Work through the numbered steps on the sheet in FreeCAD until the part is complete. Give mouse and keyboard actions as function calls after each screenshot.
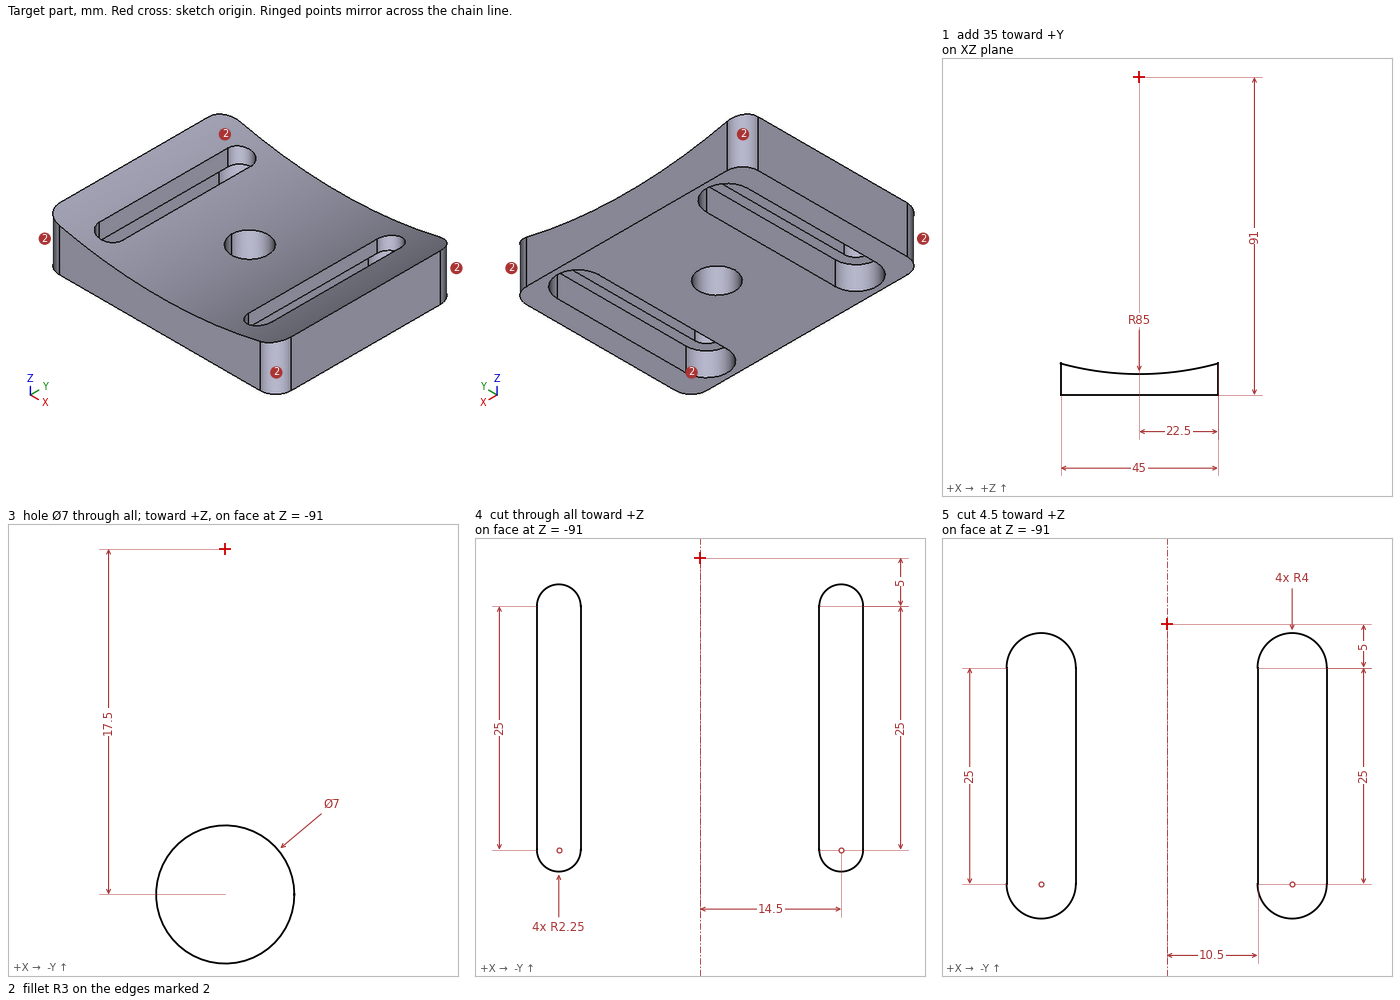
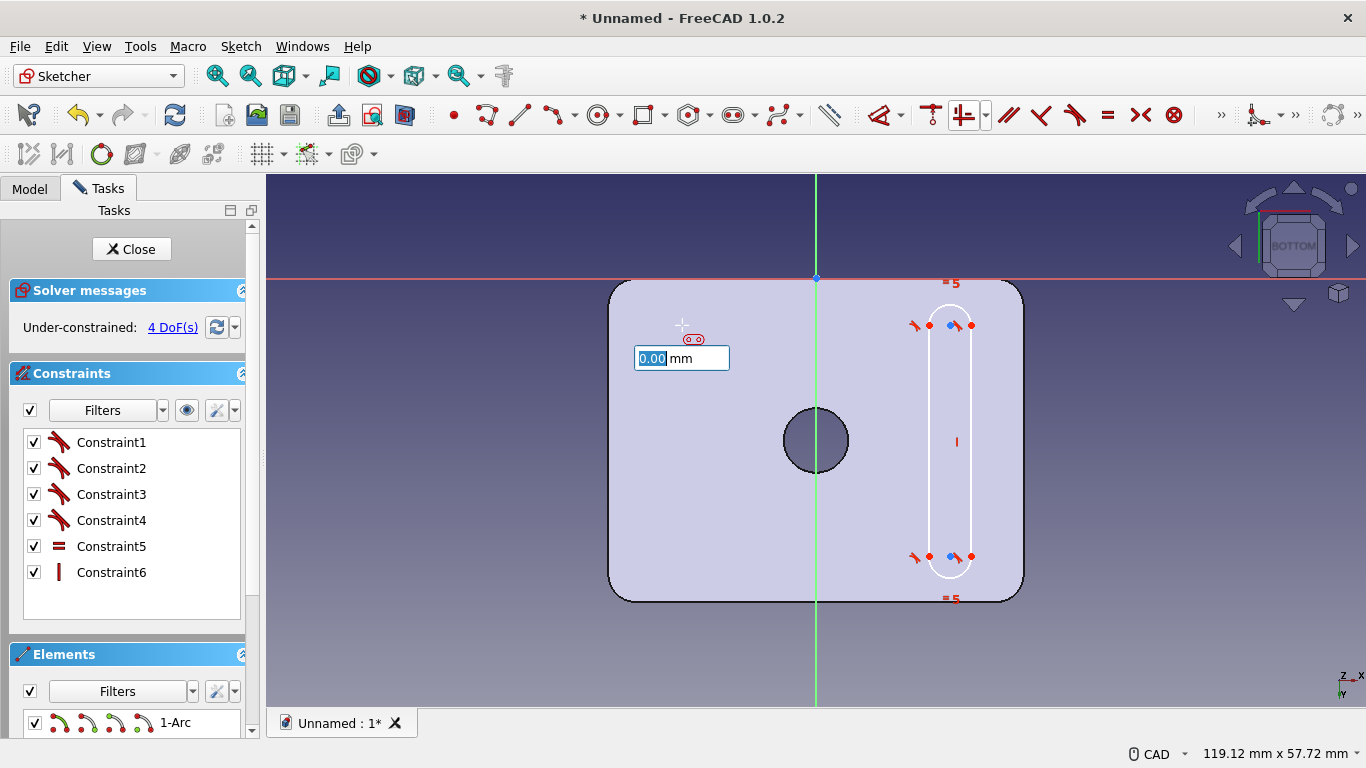
click(661, 440)
key(Escape)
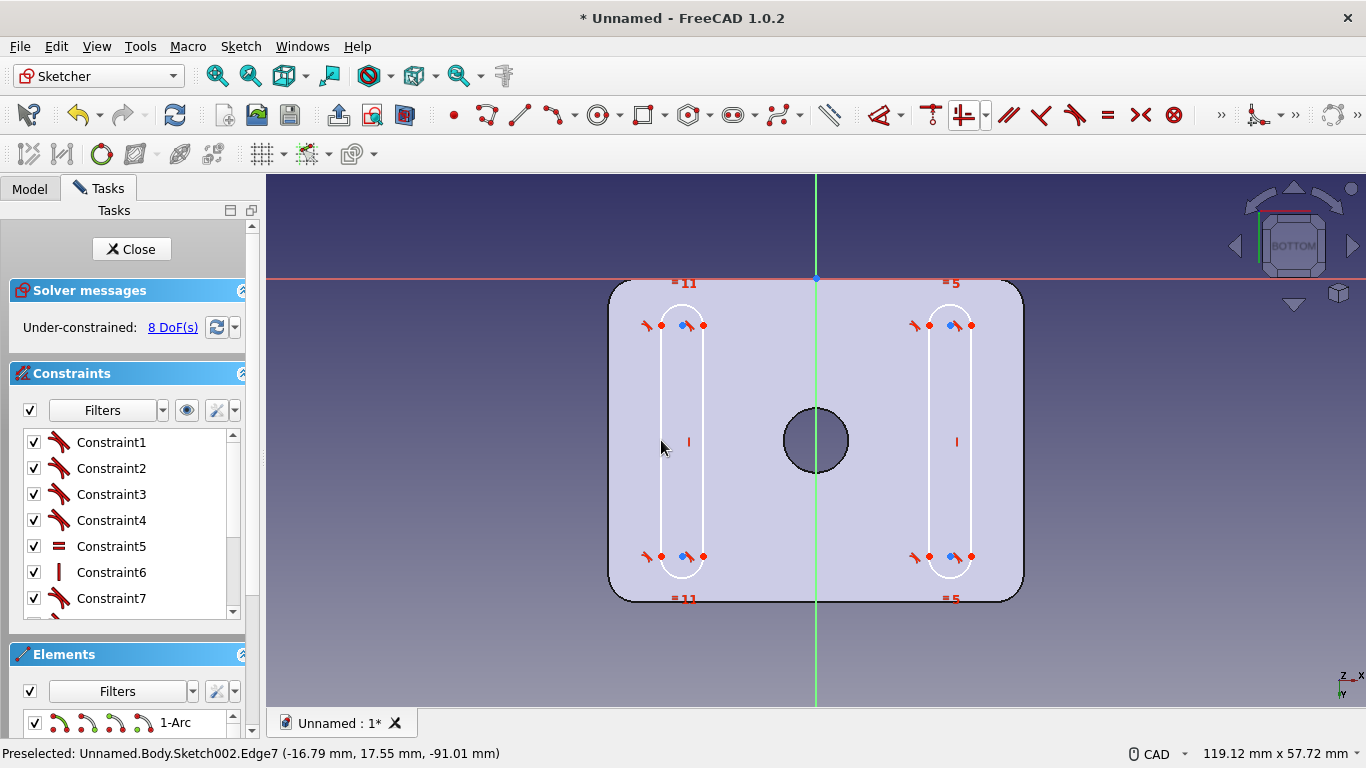
click(938, 574)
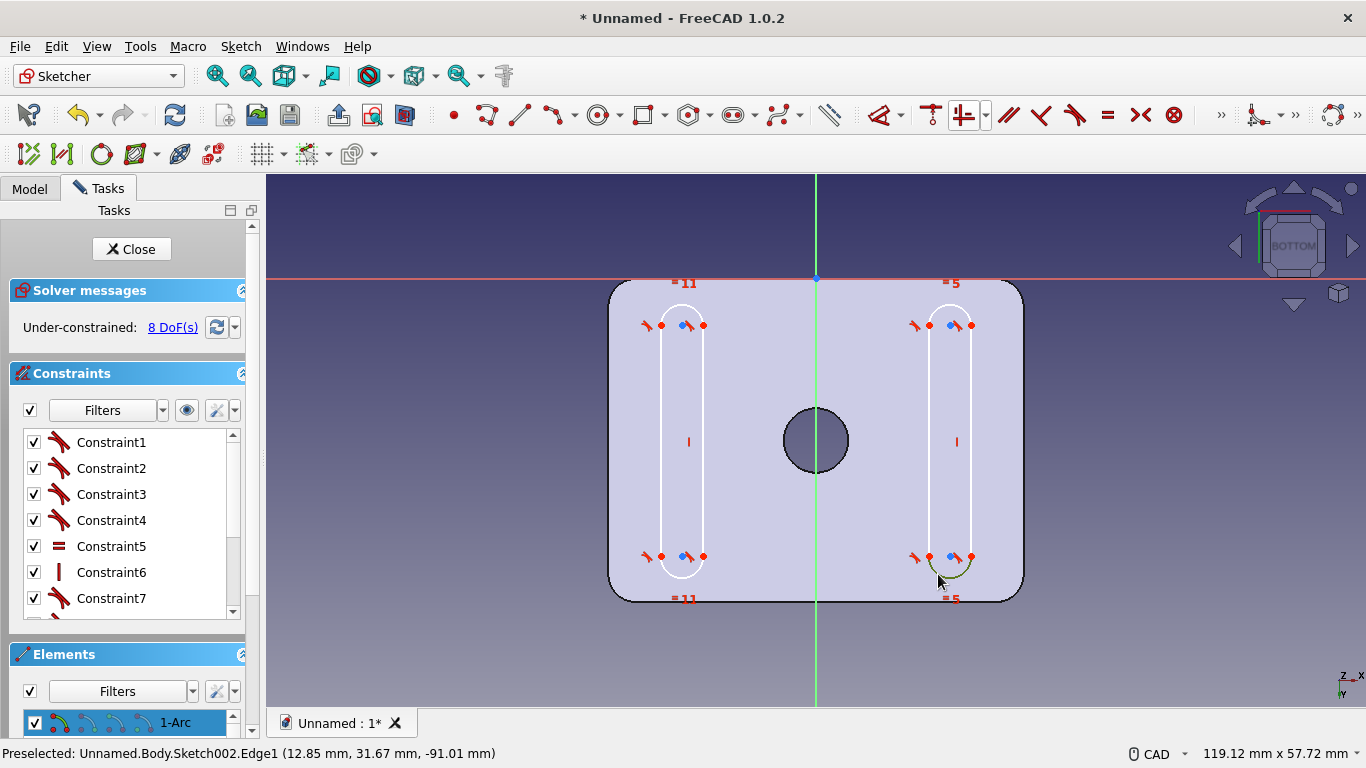
click(670, 574)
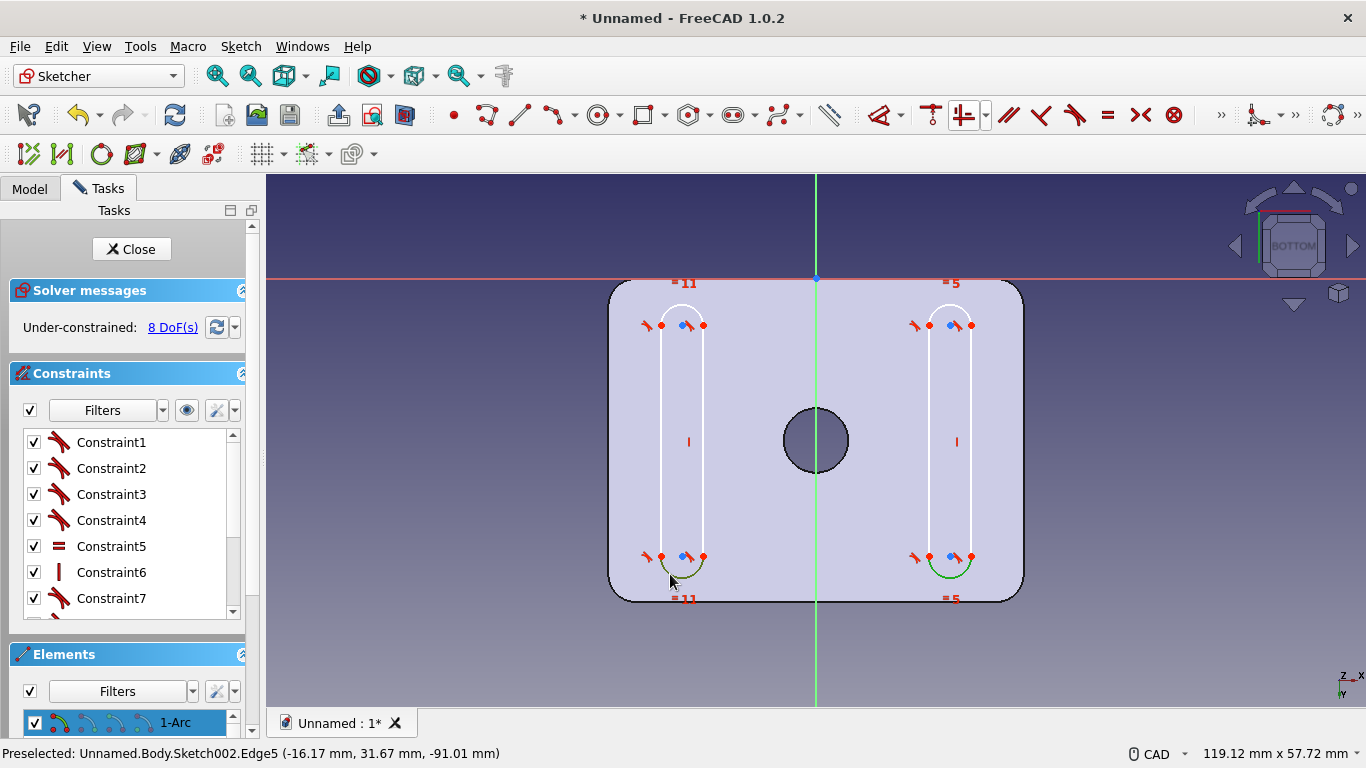
click(1108, 116)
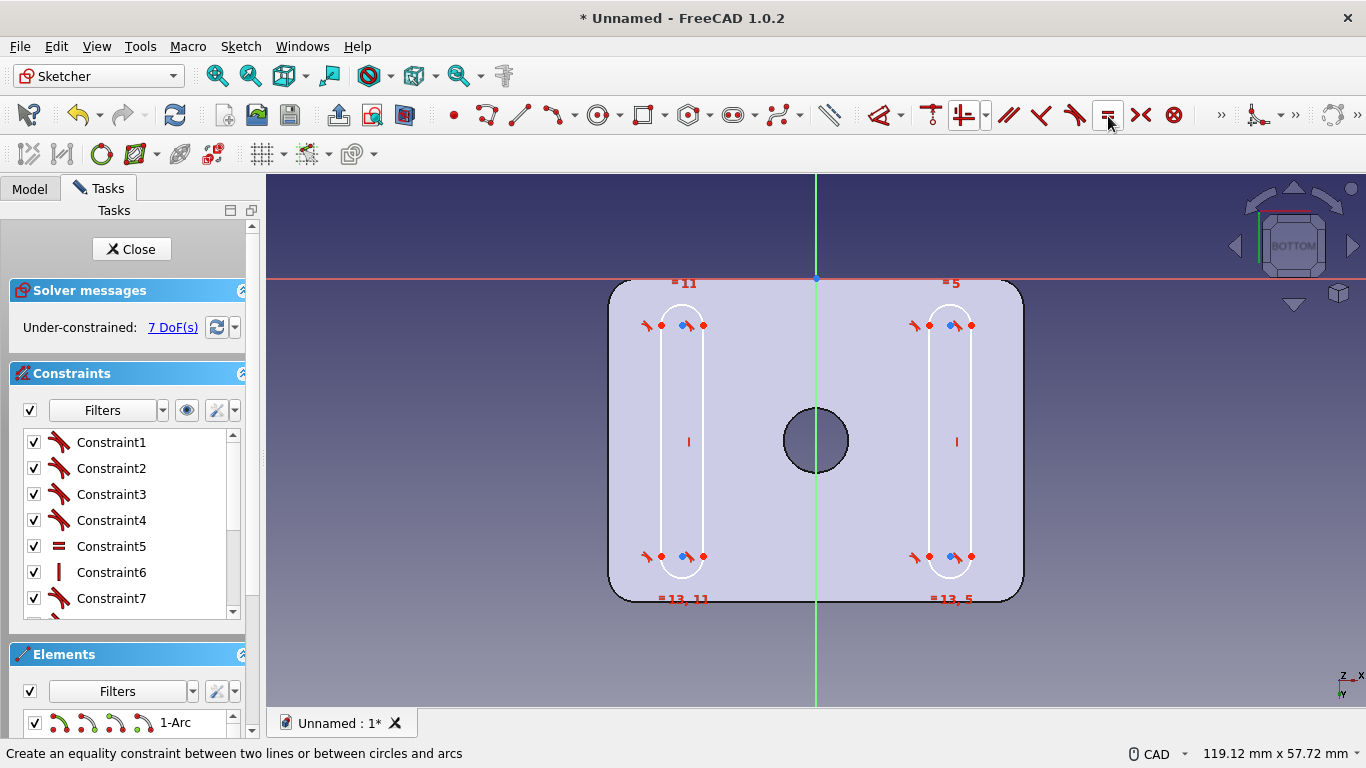
click(950, 557)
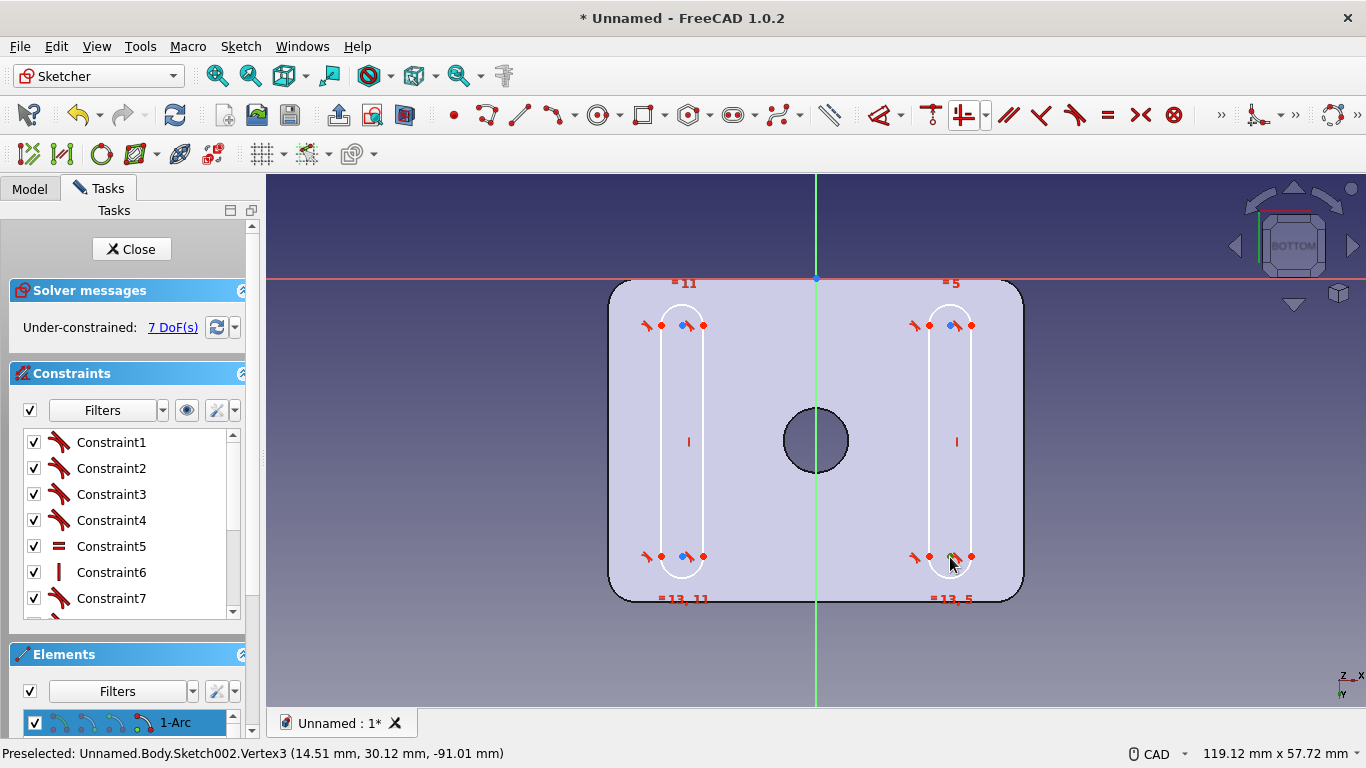
click(682, 557)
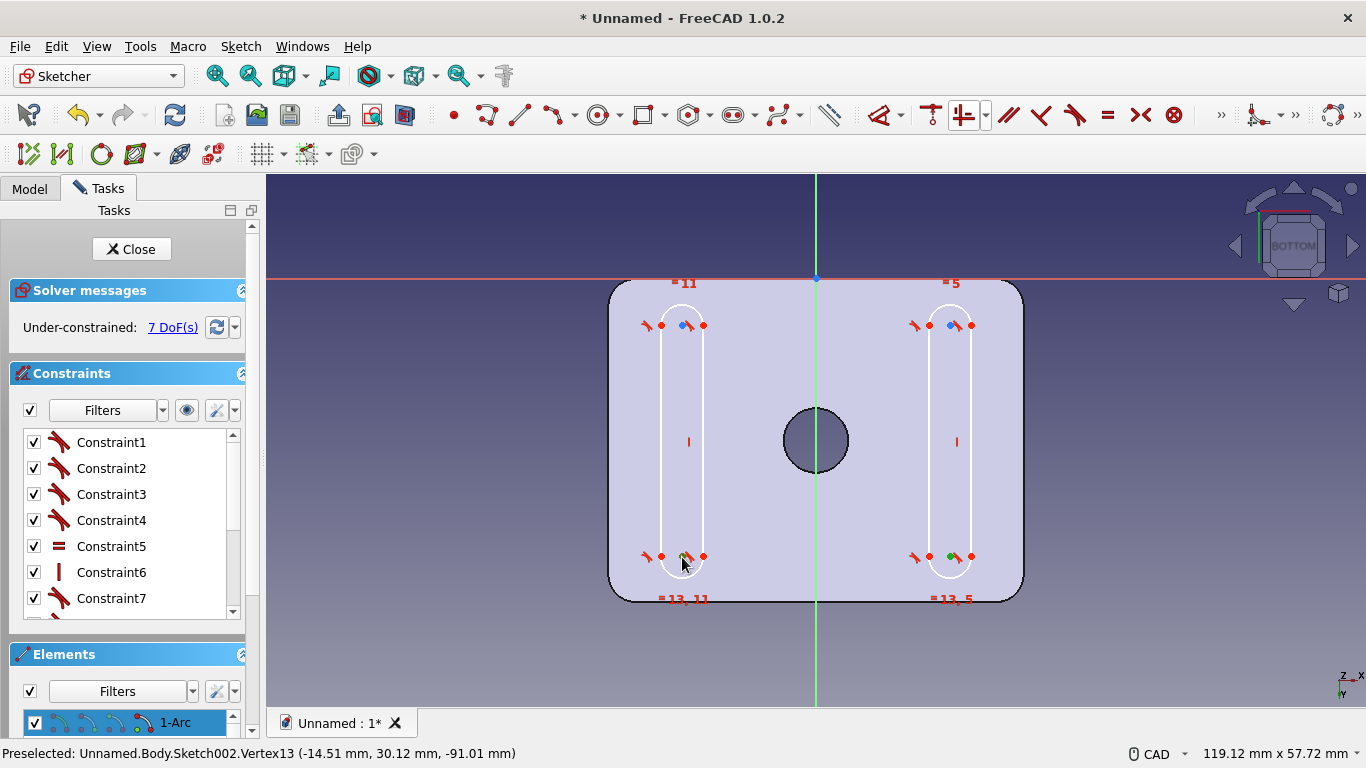
click(816, 645)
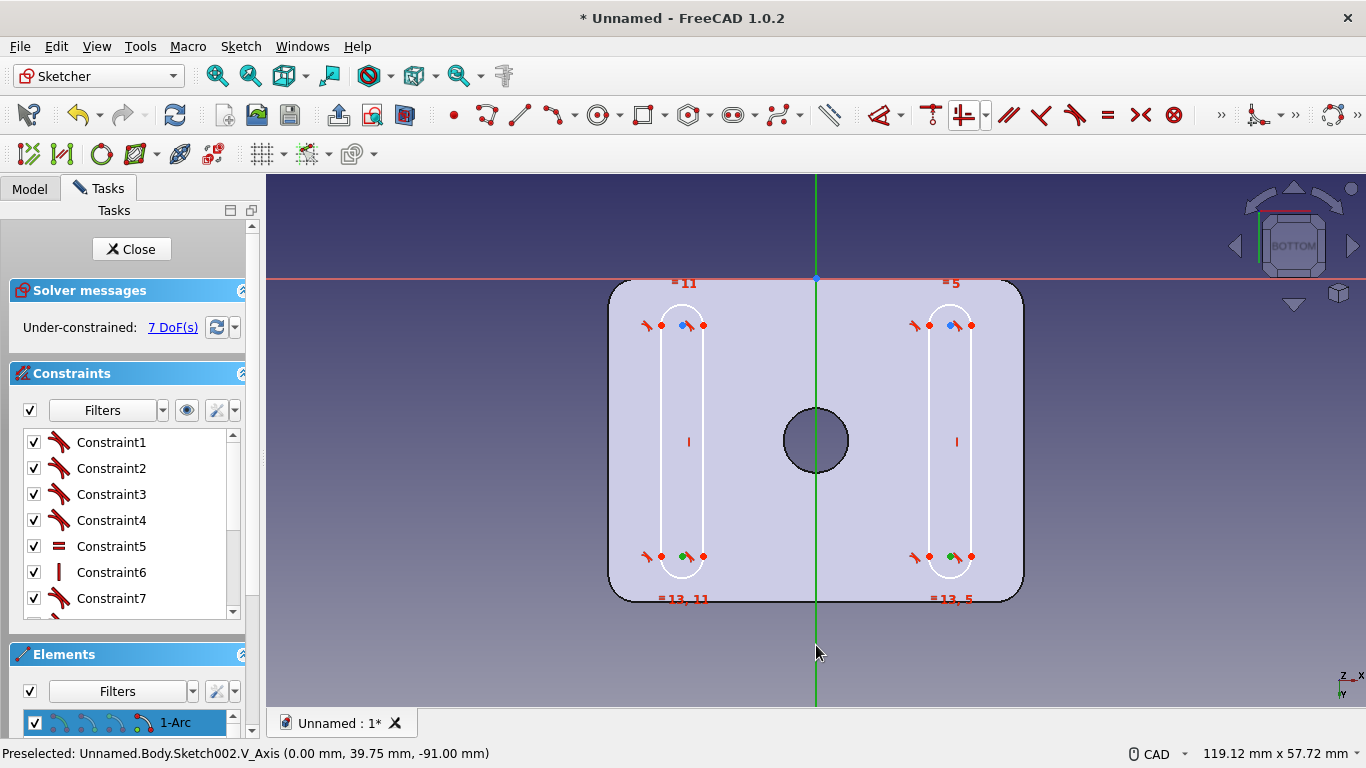
key(s)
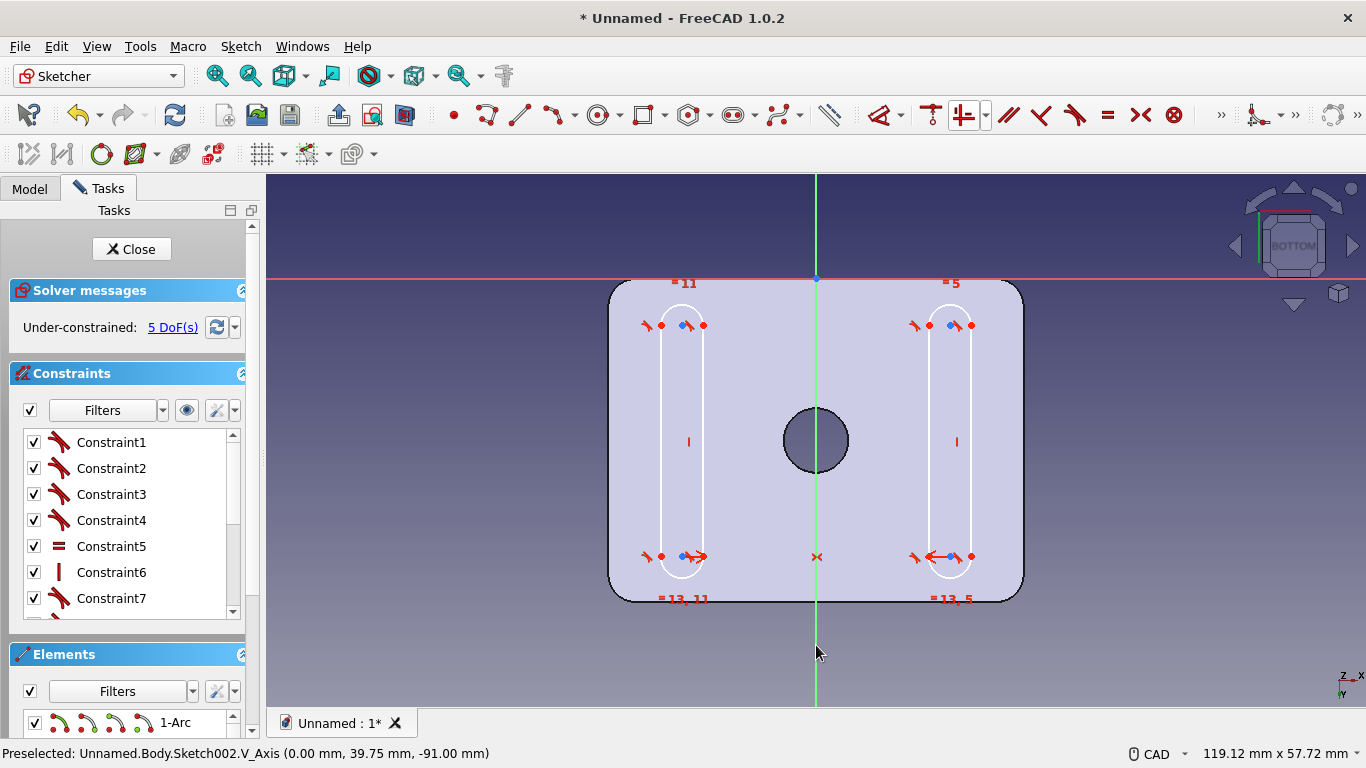
key(d)